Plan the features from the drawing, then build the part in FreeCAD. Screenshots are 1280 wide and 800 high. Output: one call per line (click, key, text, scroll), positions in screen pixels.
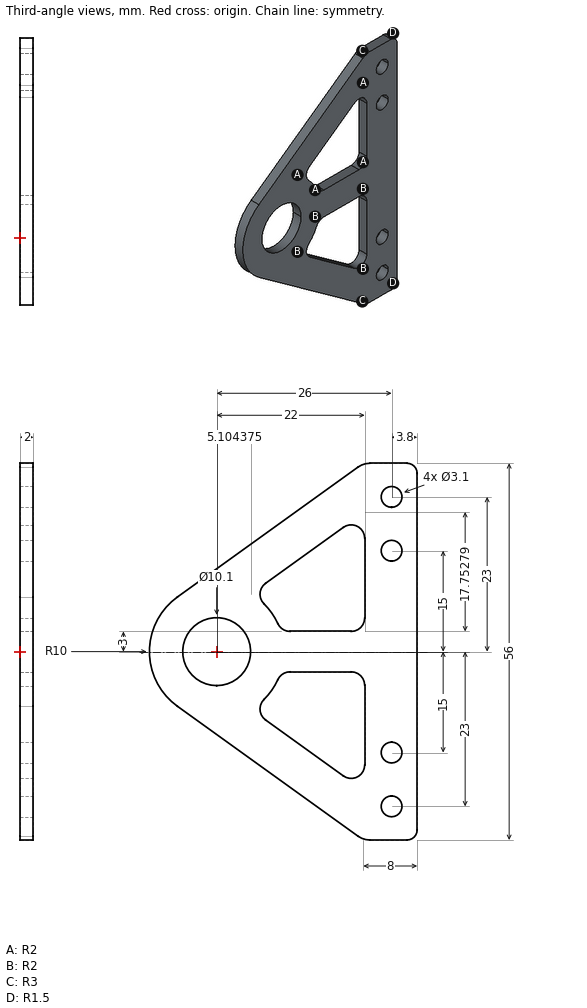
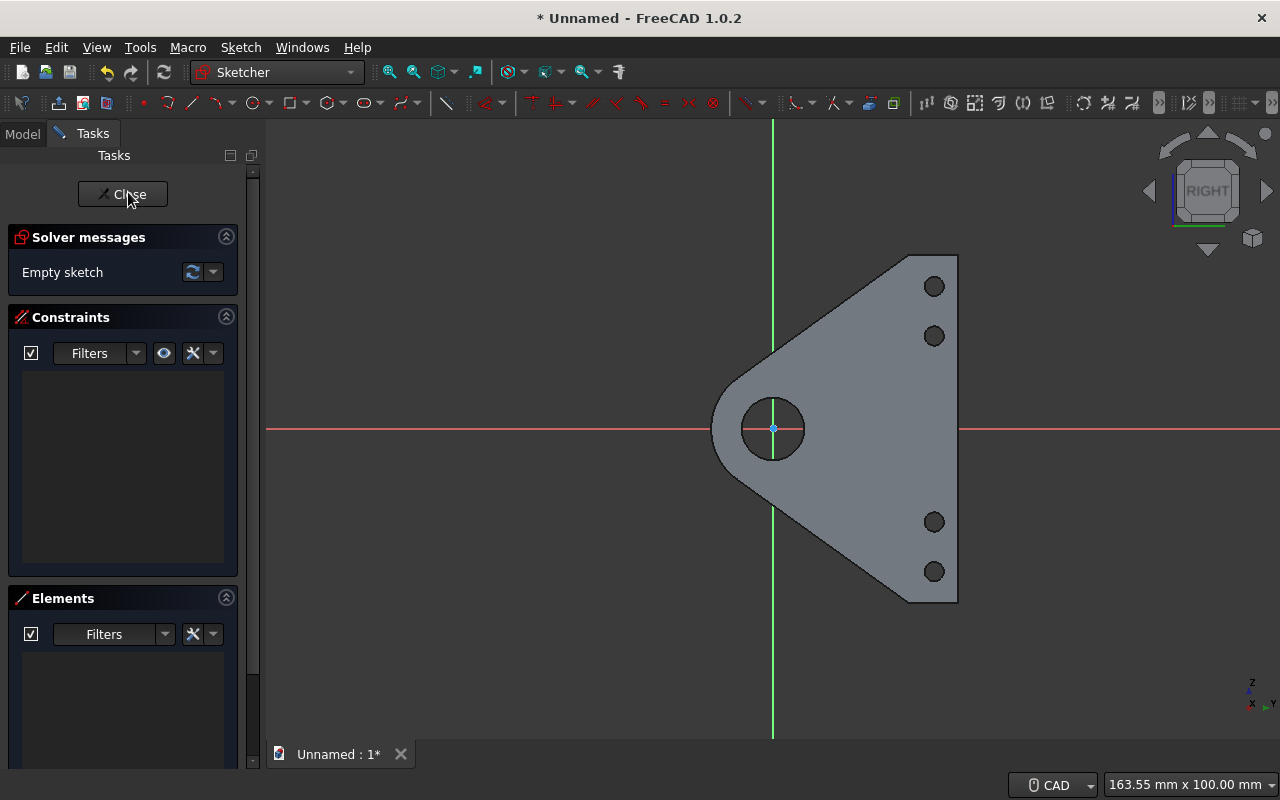
click(108, 104)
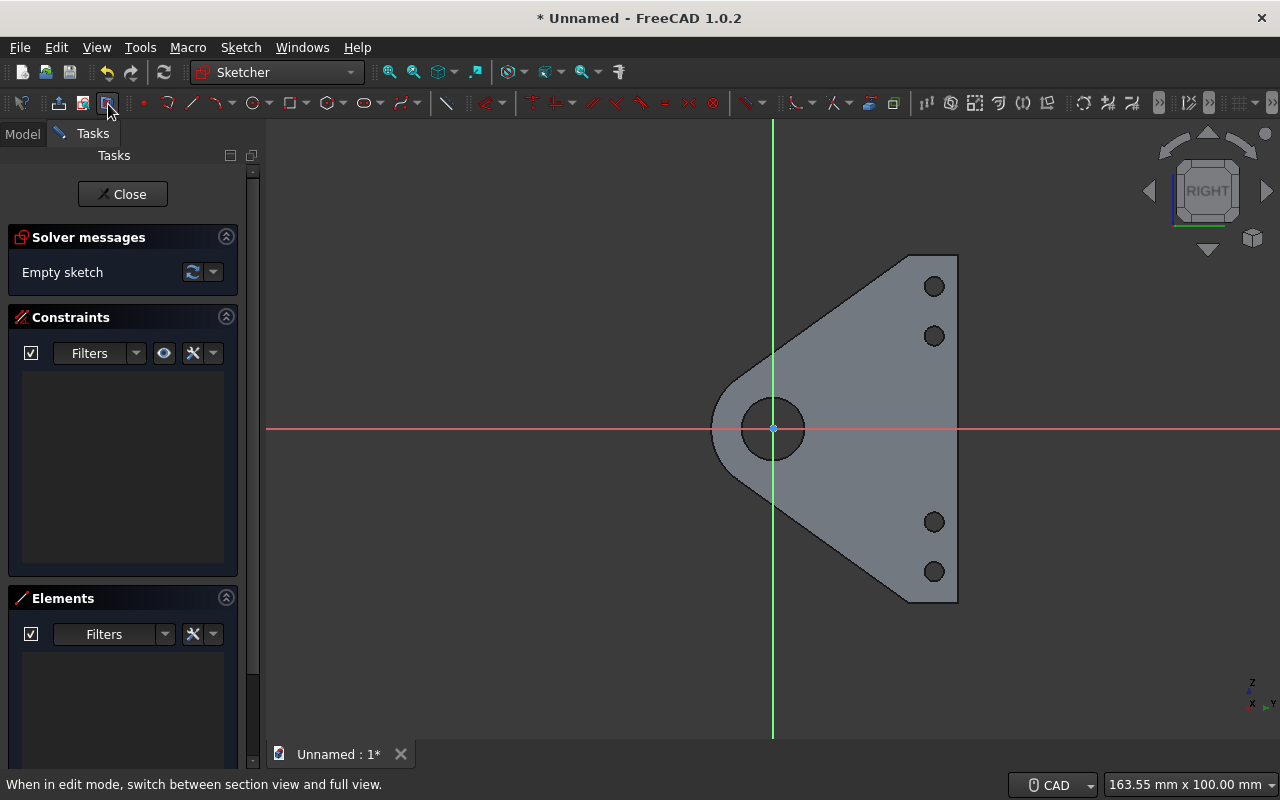
scroll(900, 337, up, 6)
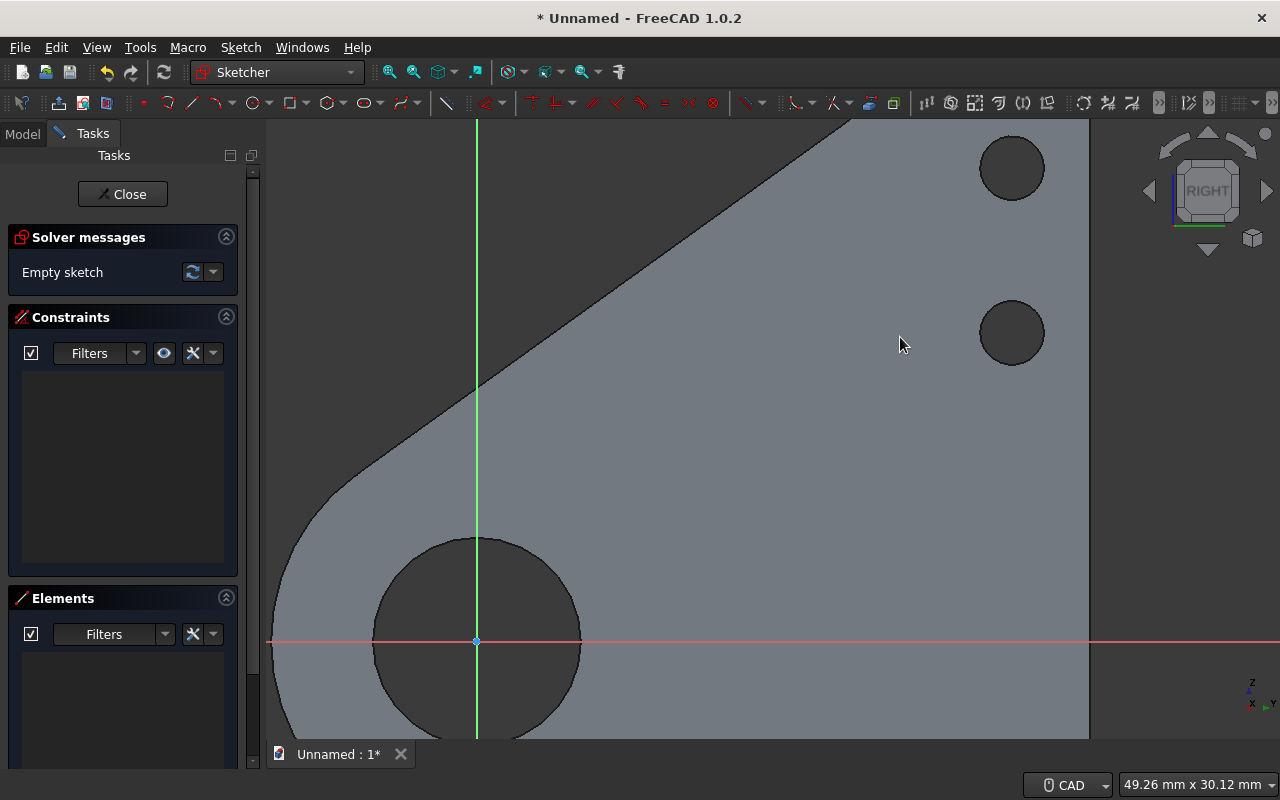
click(168, 104)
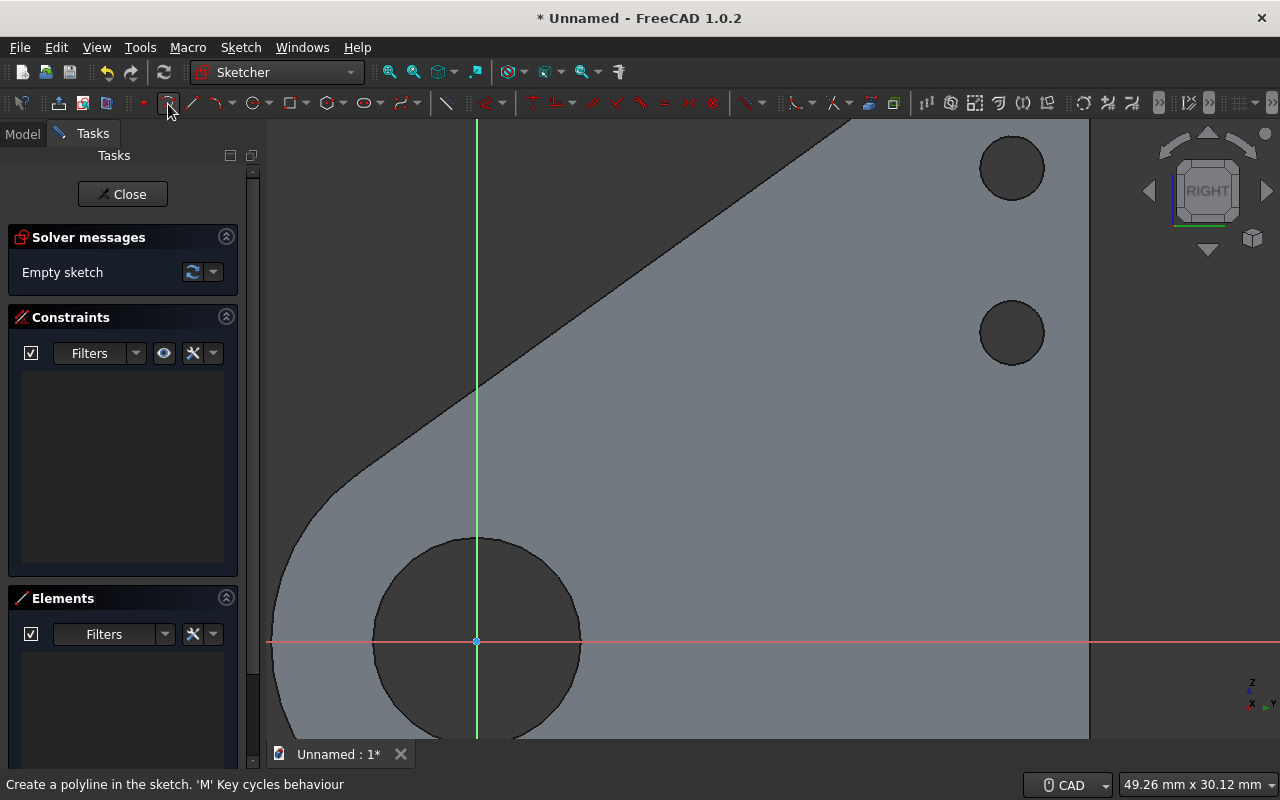
click(673, 580)
click(930, 580)
click(930, 214)
click(582, 465)
right_click(582, 465)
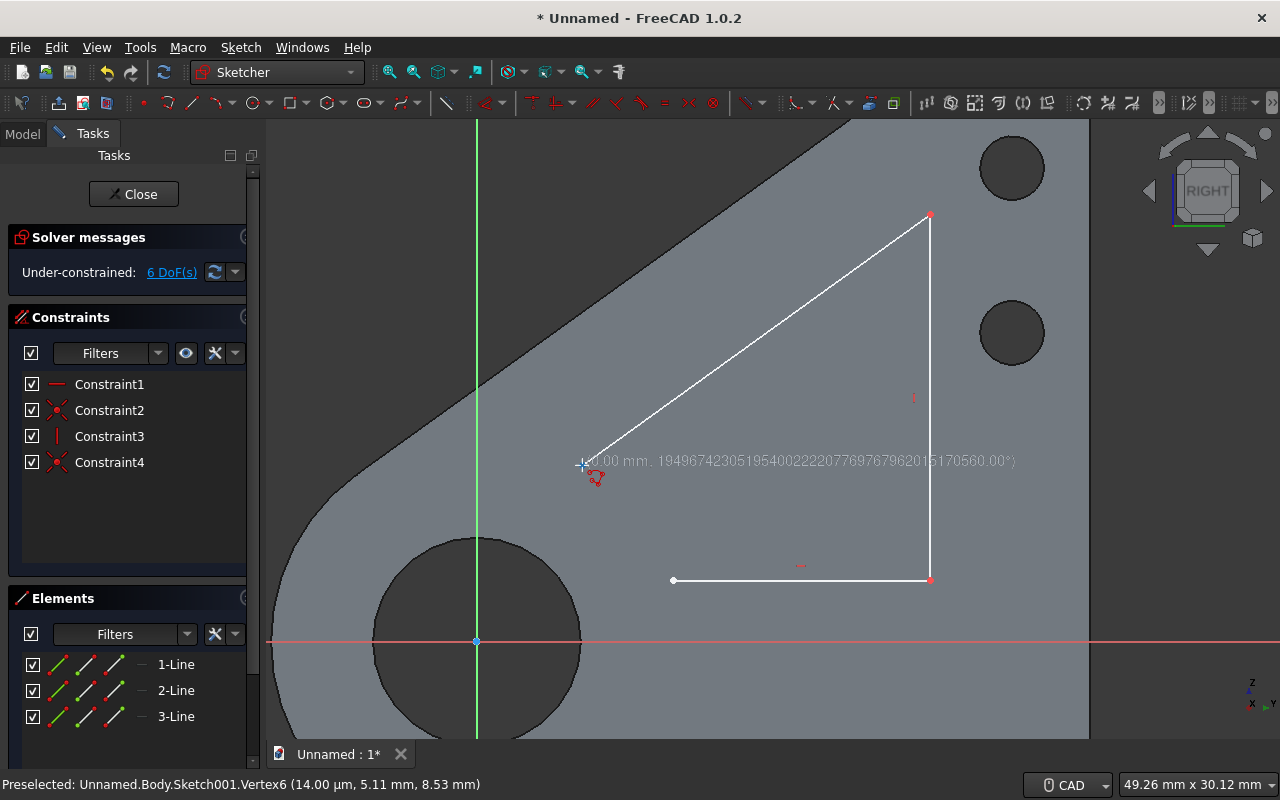
click(216, 104)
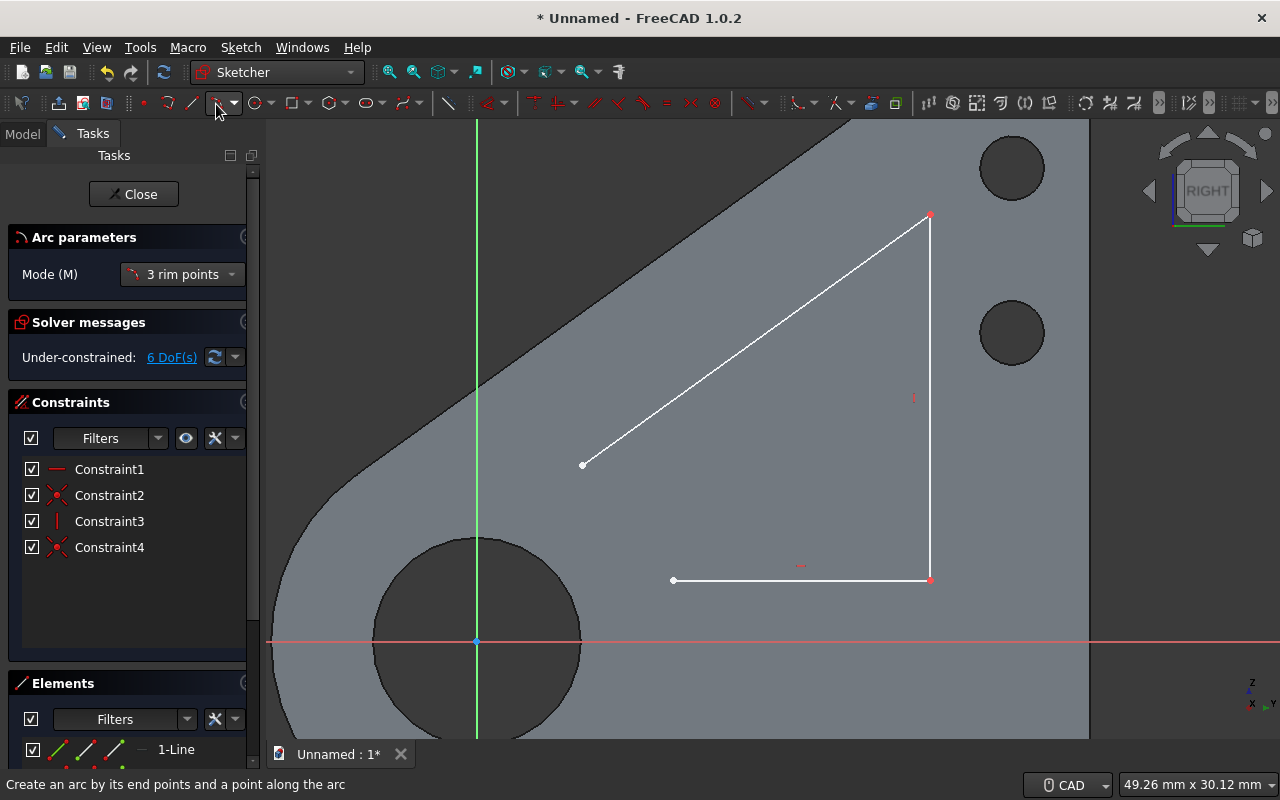
click(582, 466)
click(673, 581)
click(638, 514)
key(Escape)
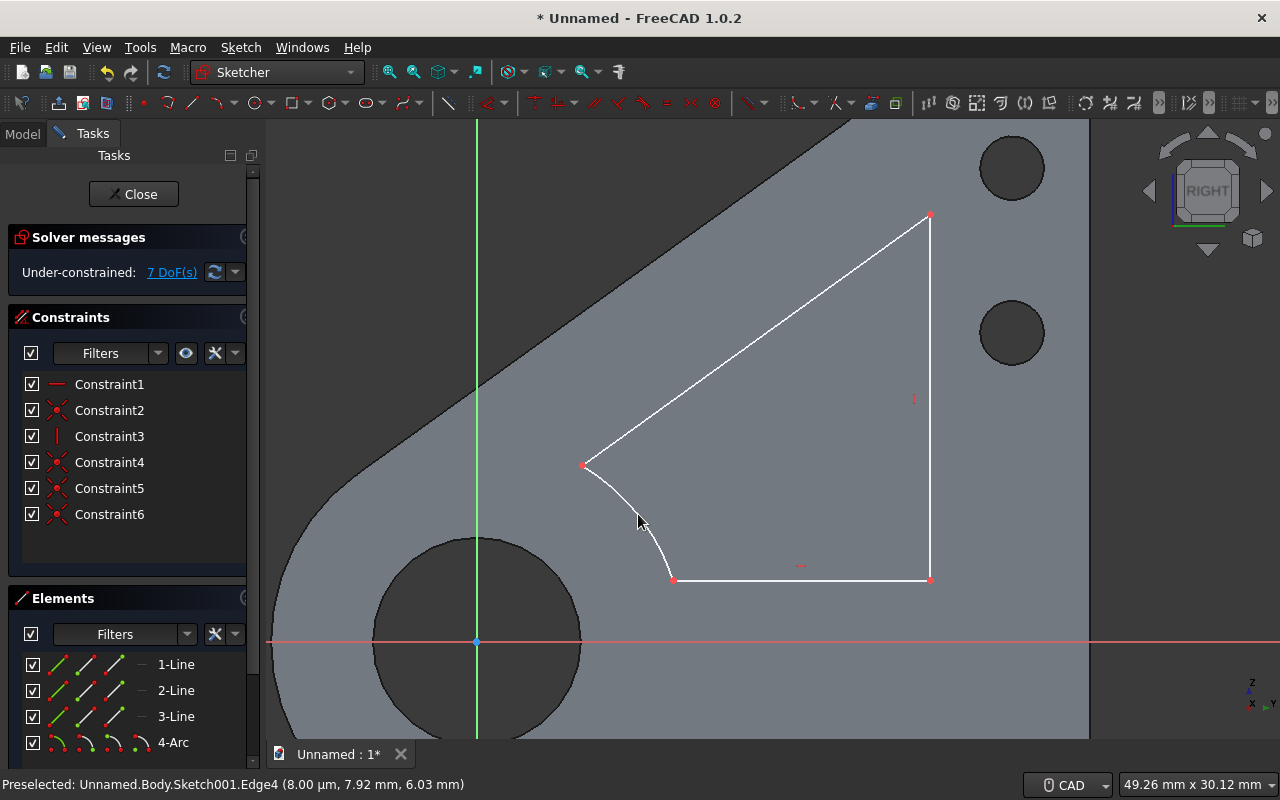
drag(467, 632, 487, 653)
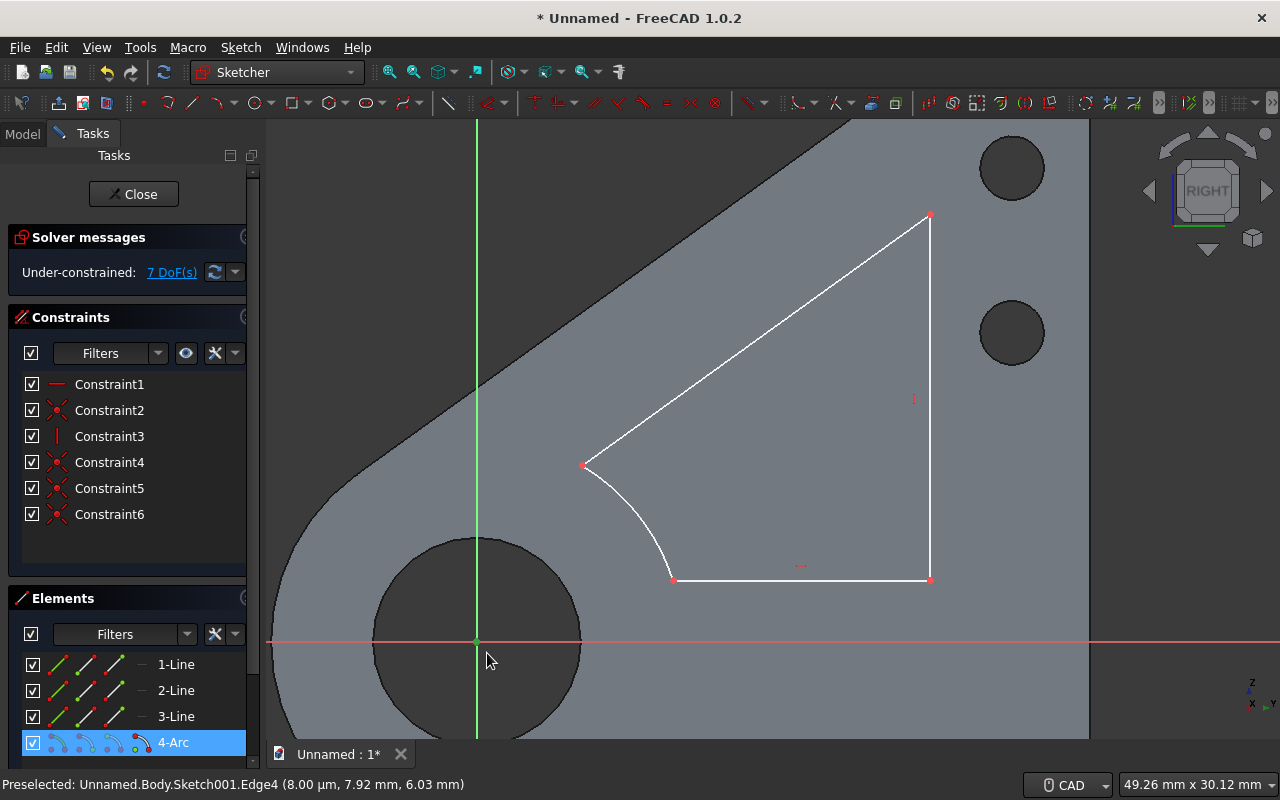
click(534, 104)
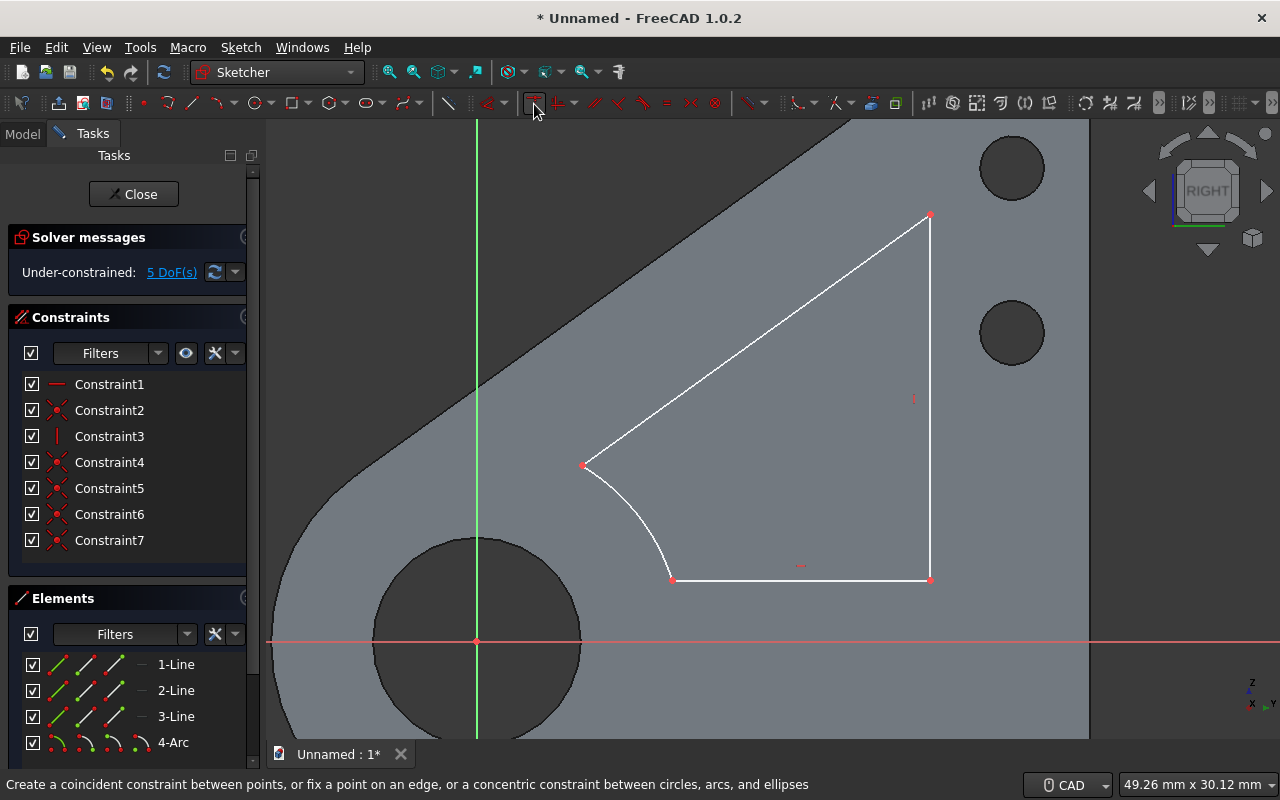
click(488, 104)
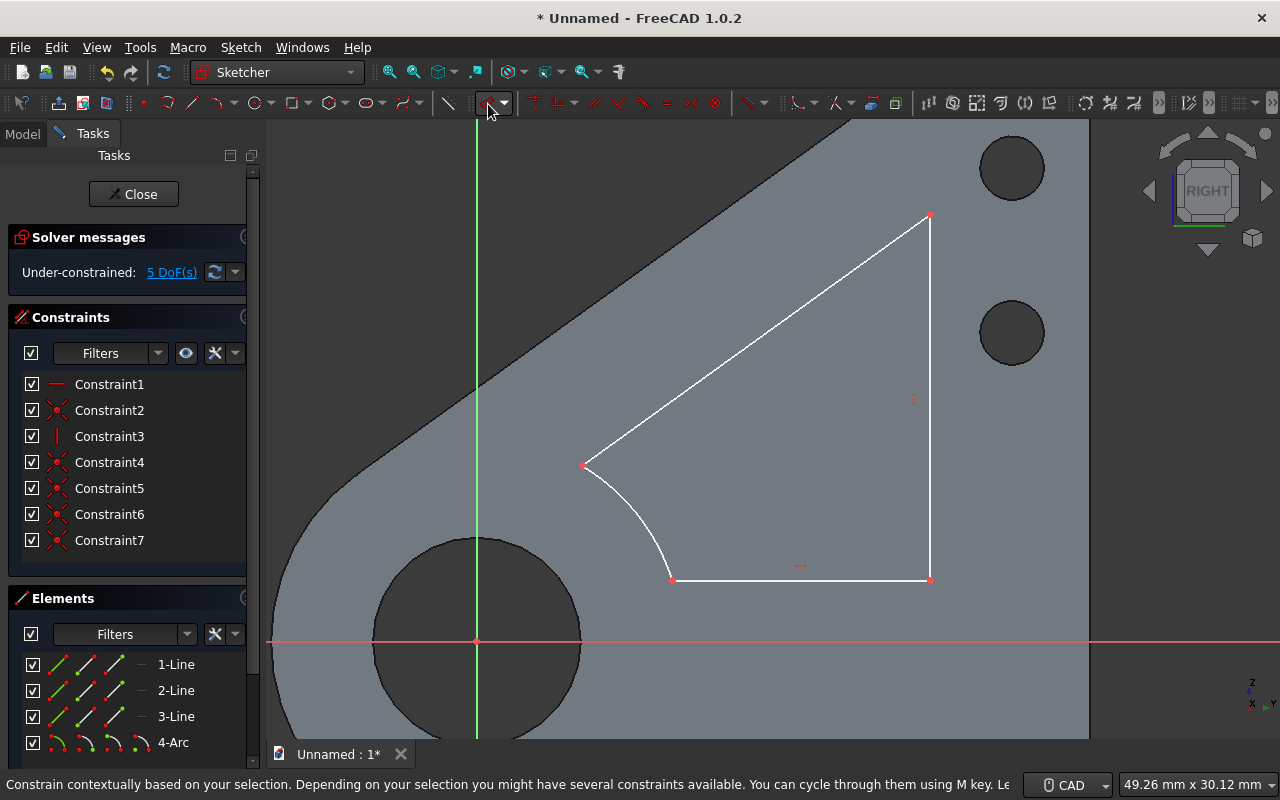
click(655, 540)
click(683, 524)